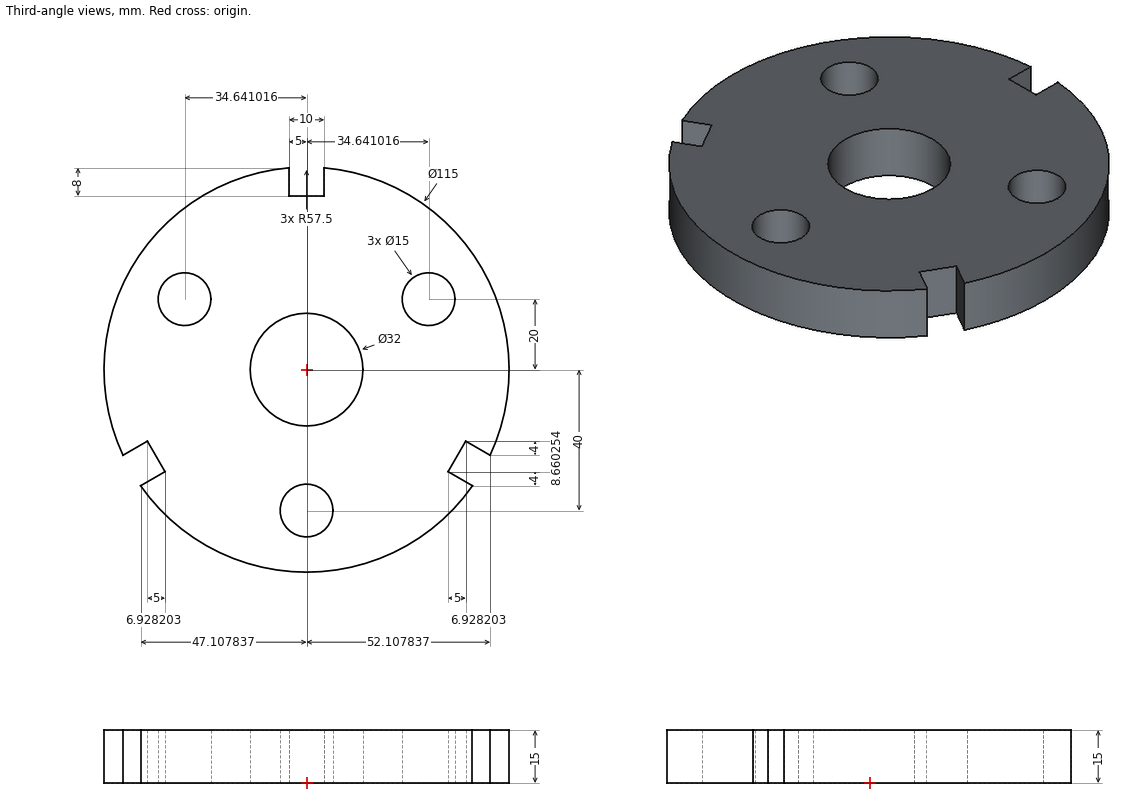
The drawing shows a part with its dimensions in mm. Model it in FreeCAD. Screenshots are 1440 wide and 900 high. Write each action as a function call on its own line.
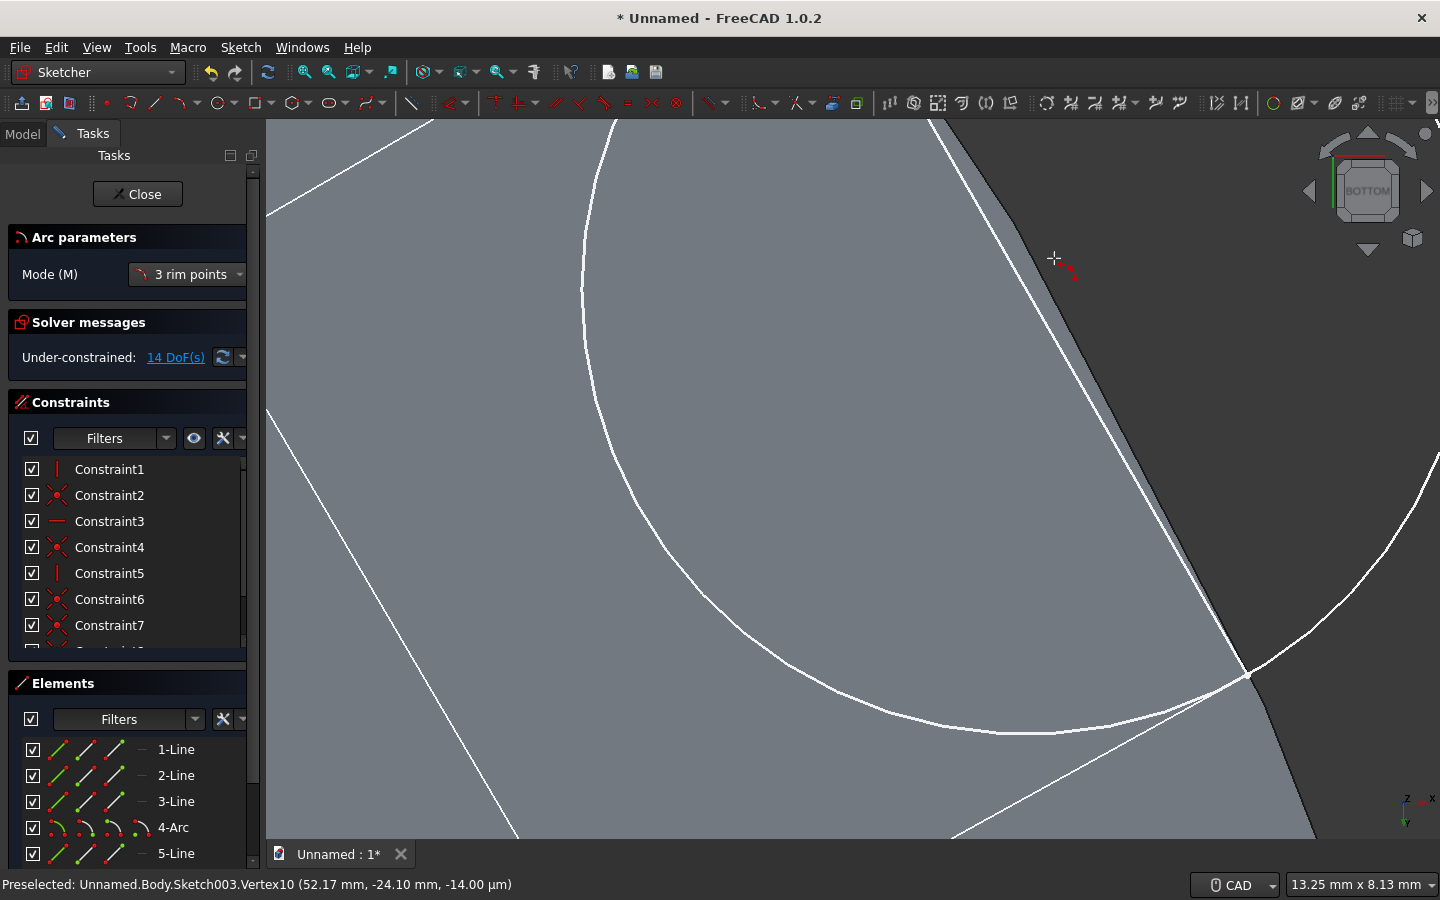
click(1037, 263)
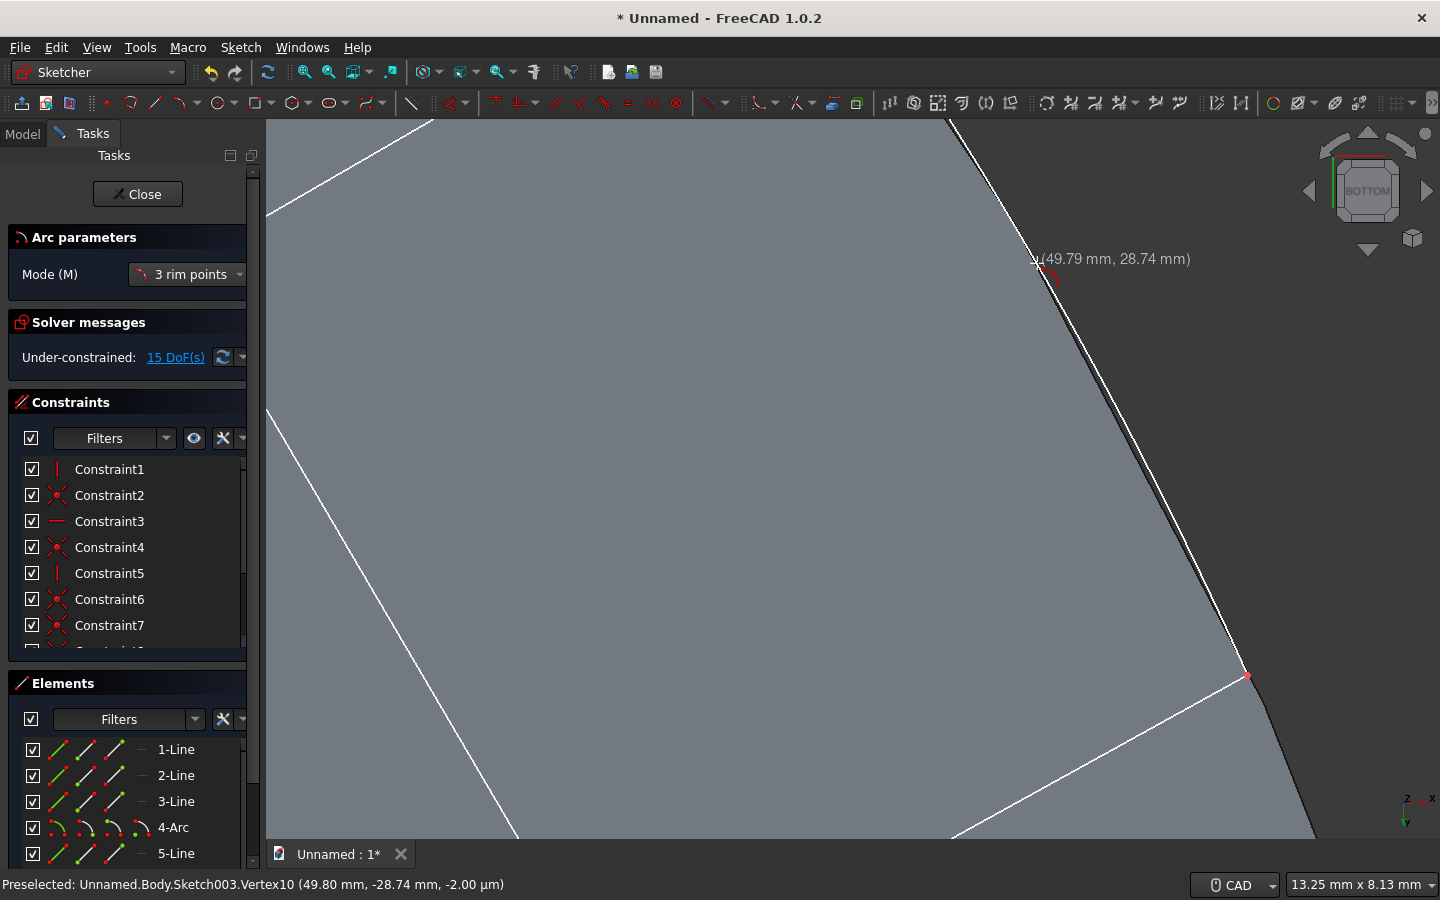
click(132, 104)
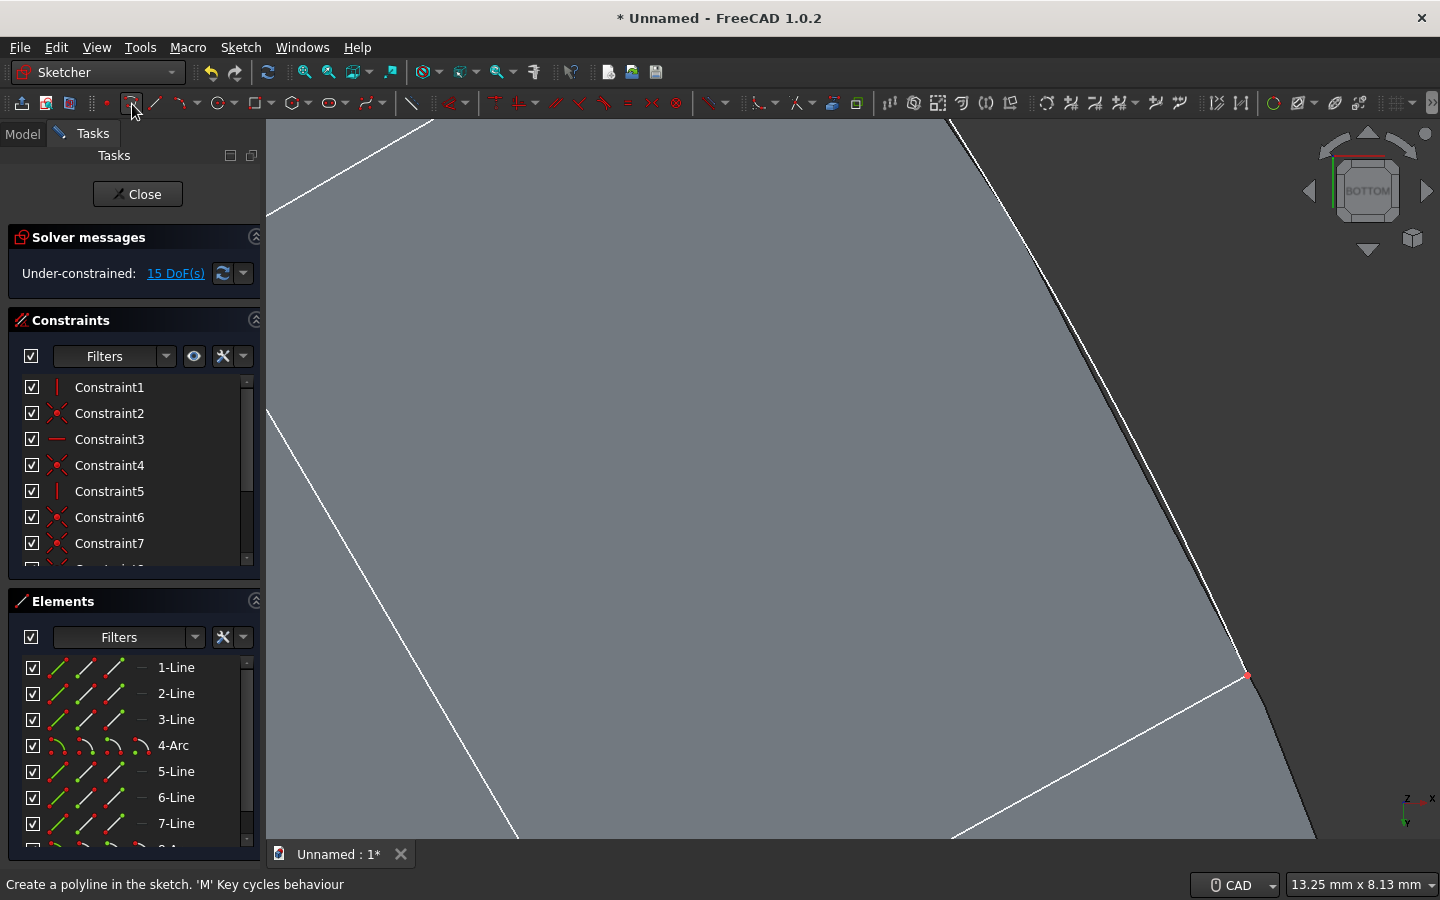
scroll(1054, 258, down, 14)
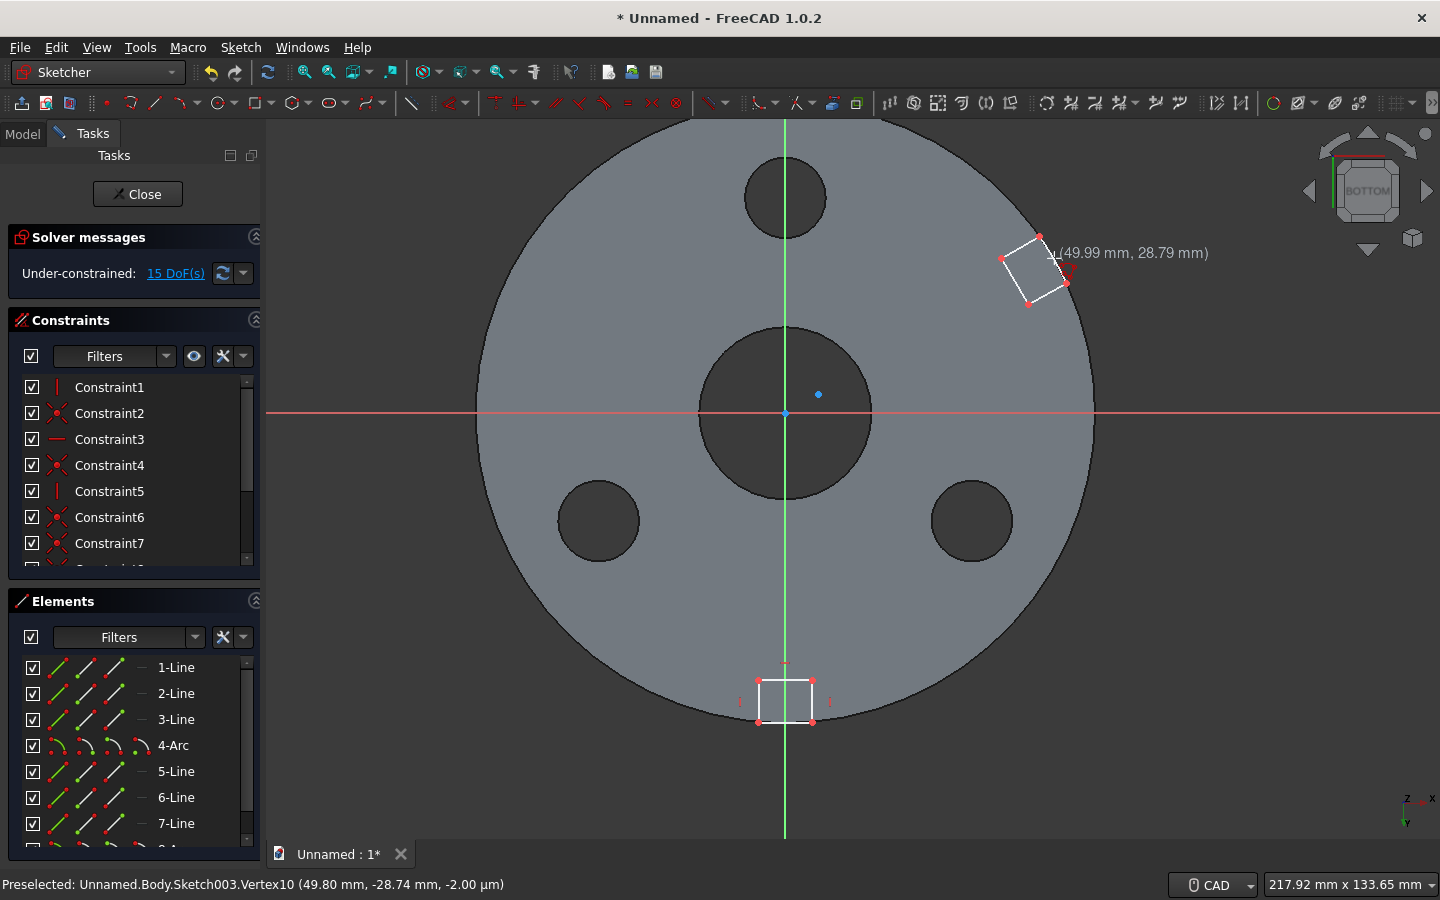
click(532, 236)
click(569, 257)
click(542, 304)
click(505, 282)
right_click(505, 282)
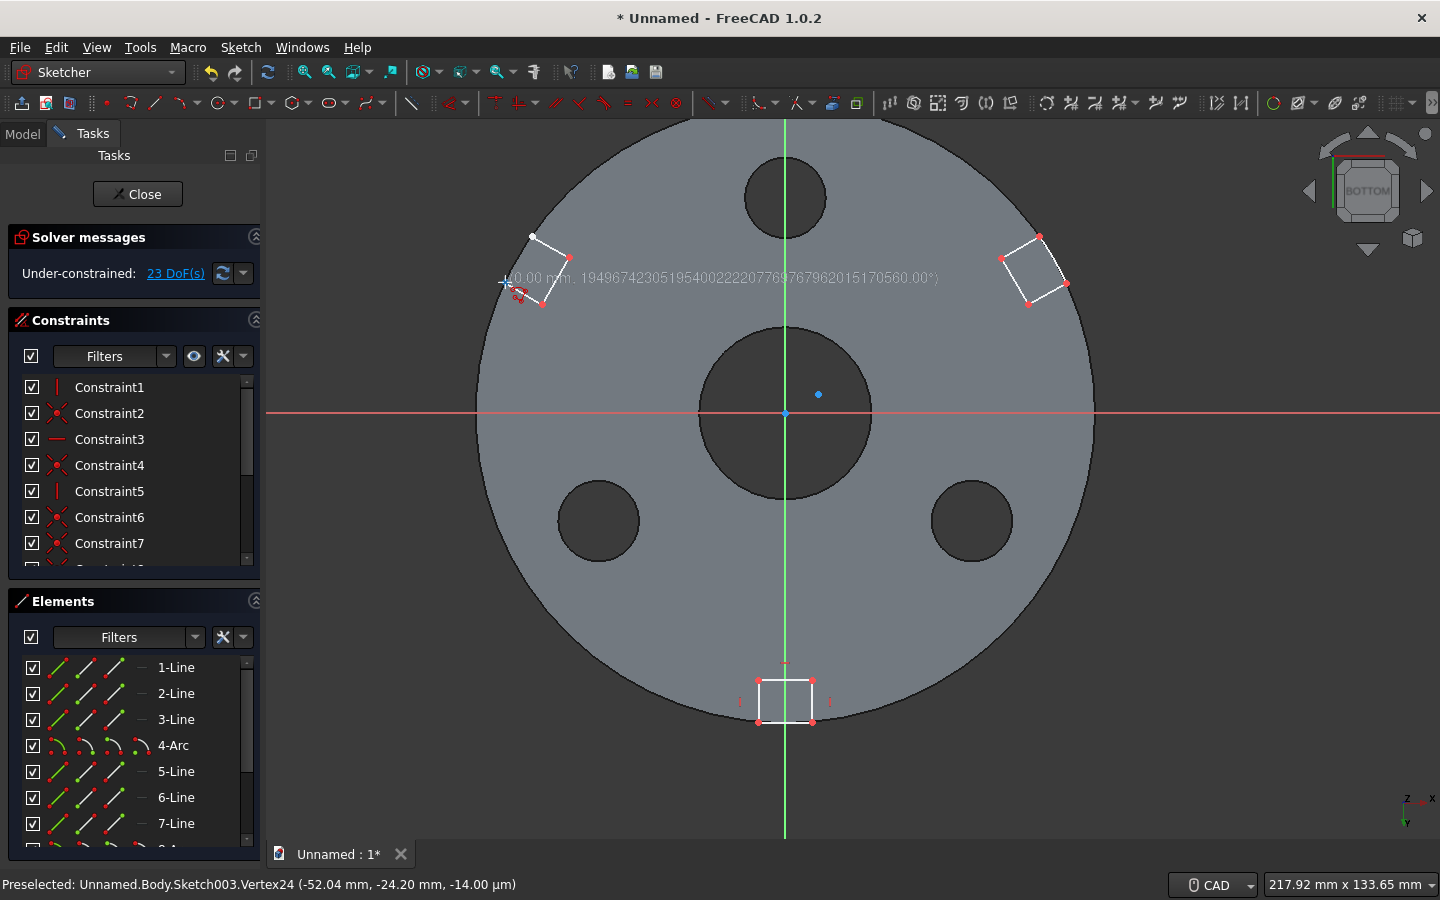
click(180, 104)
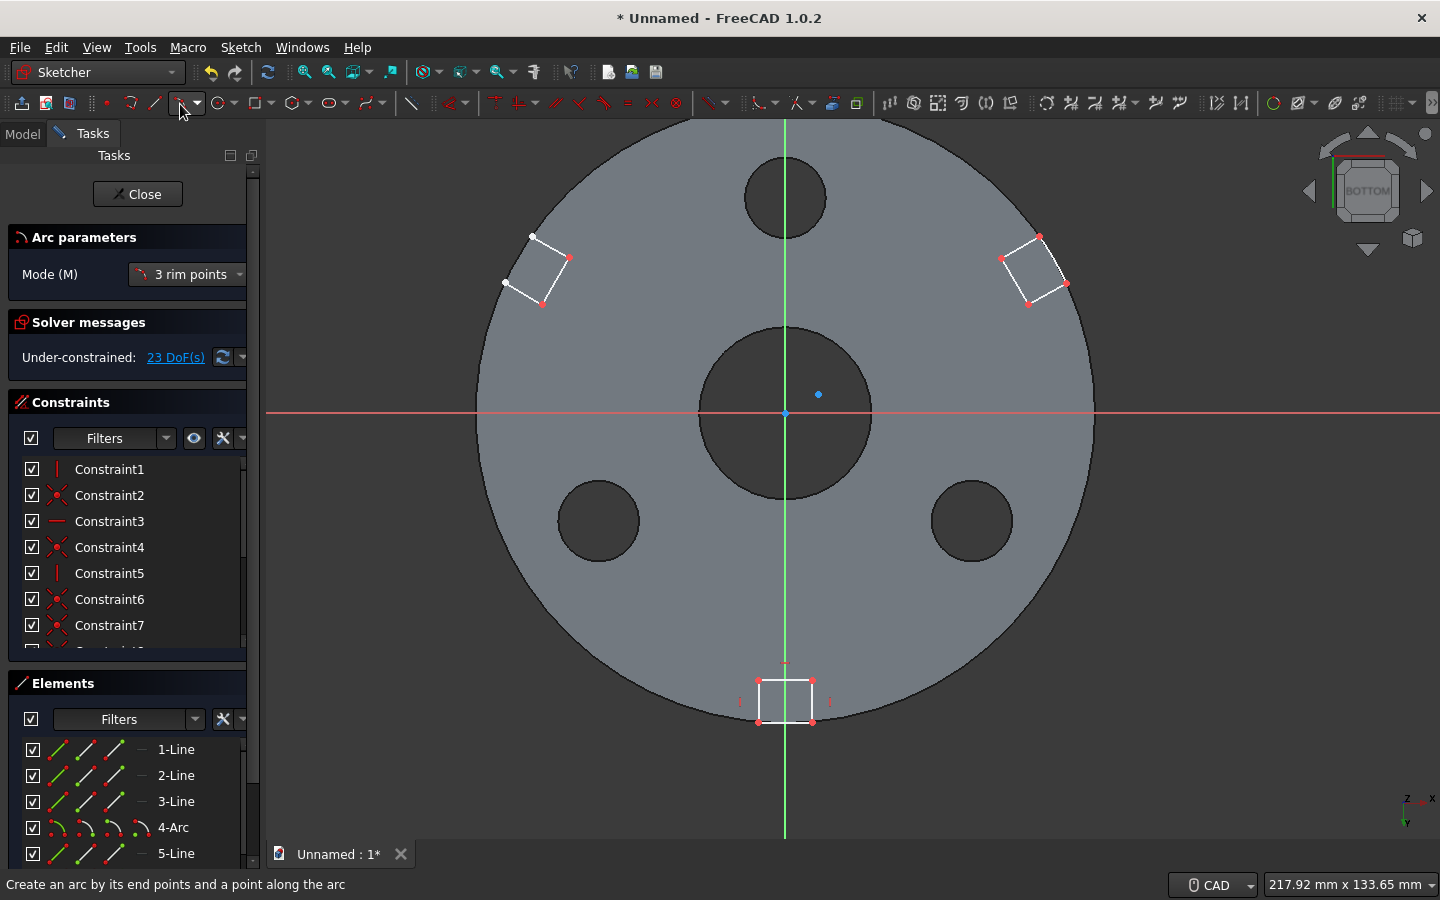
click(505, 283)
click(532, 237)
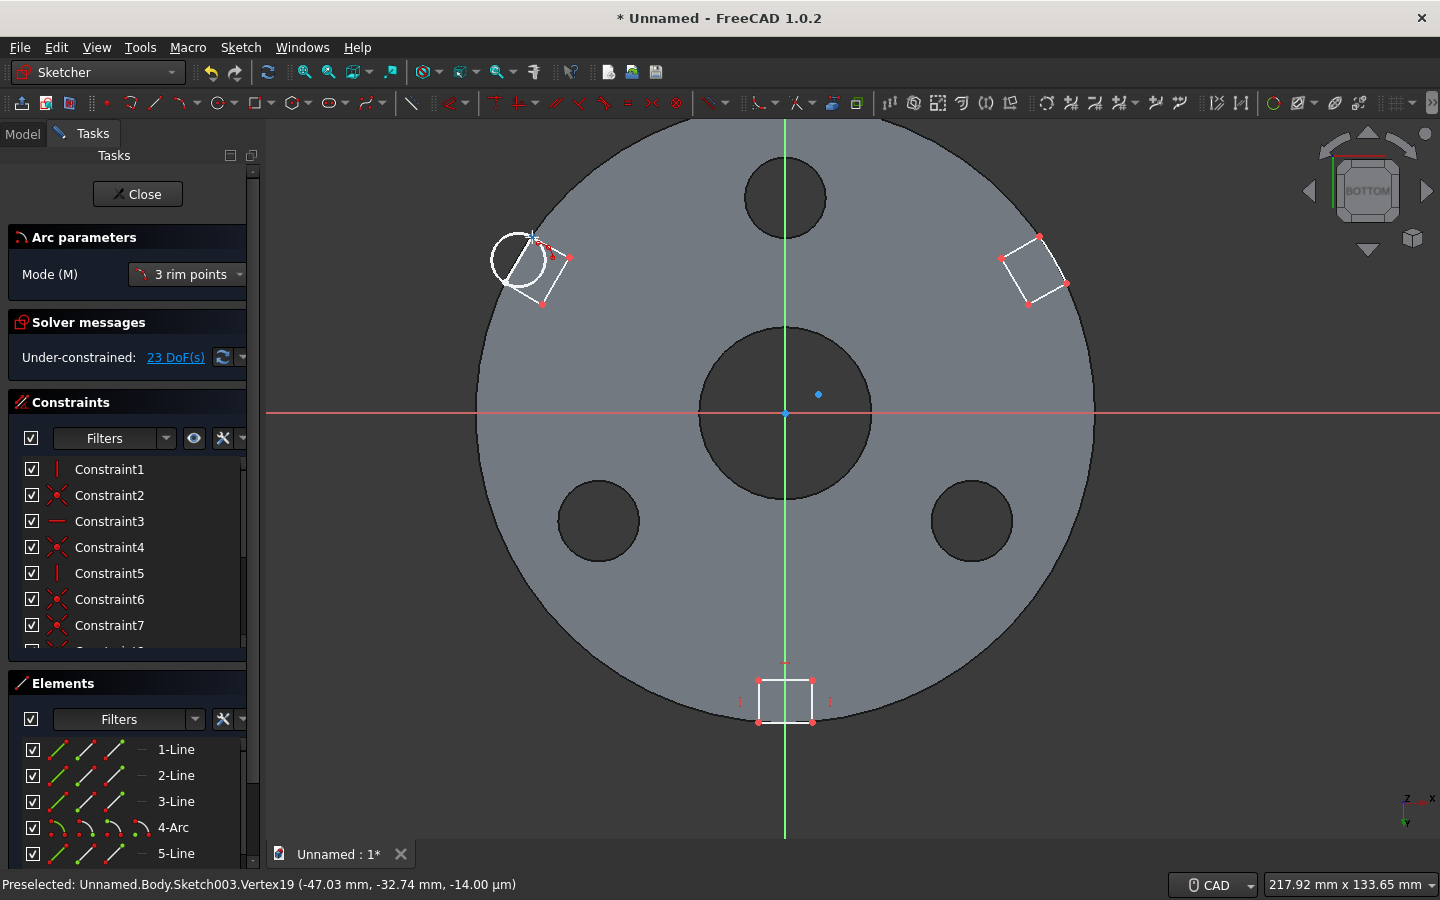
scroll(517, 258, up, 14)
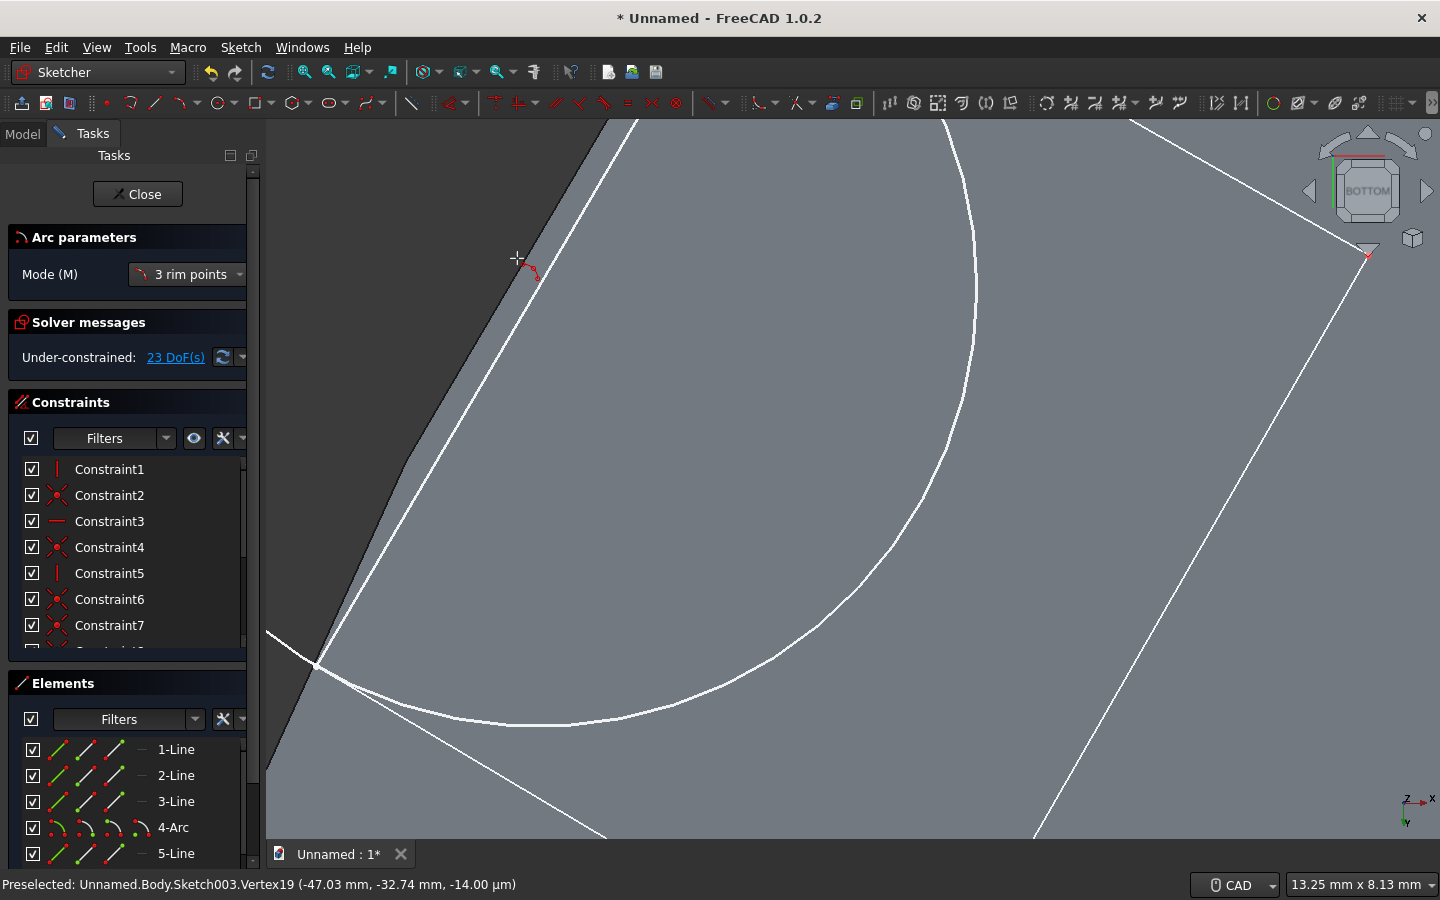
click(515, 263)
key(Escape)